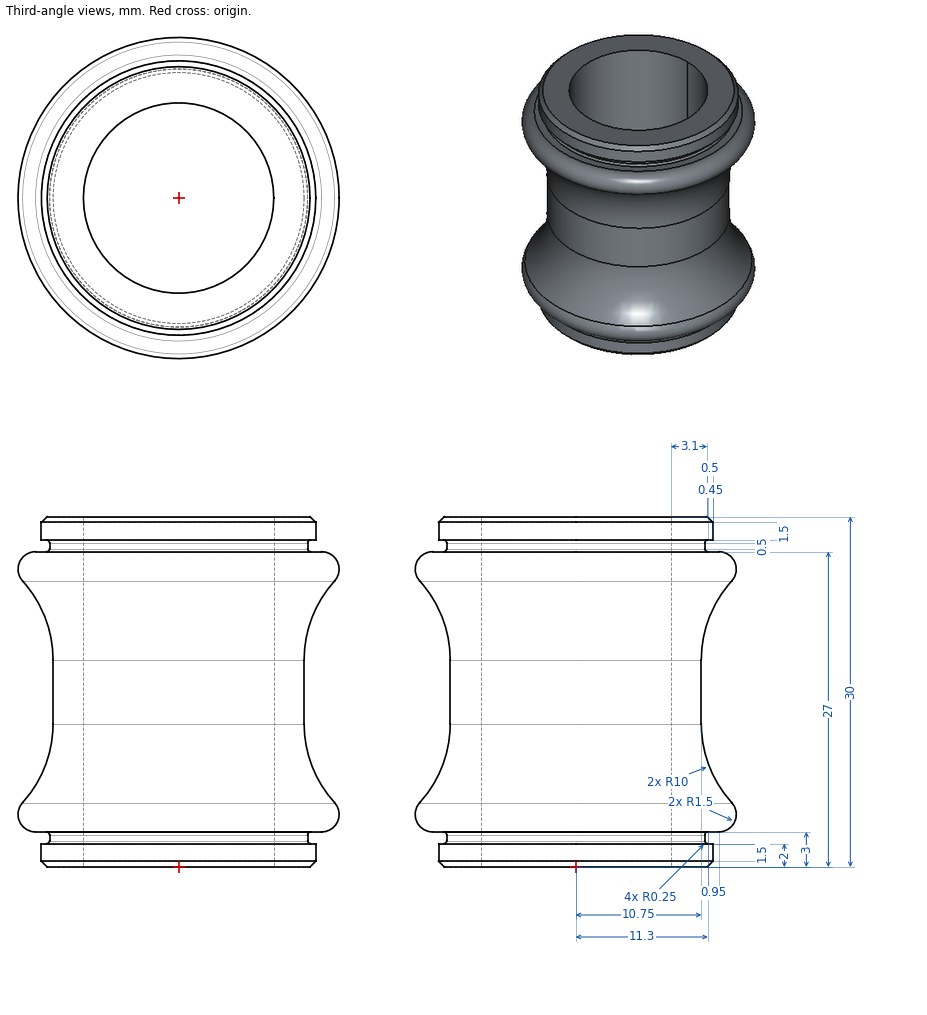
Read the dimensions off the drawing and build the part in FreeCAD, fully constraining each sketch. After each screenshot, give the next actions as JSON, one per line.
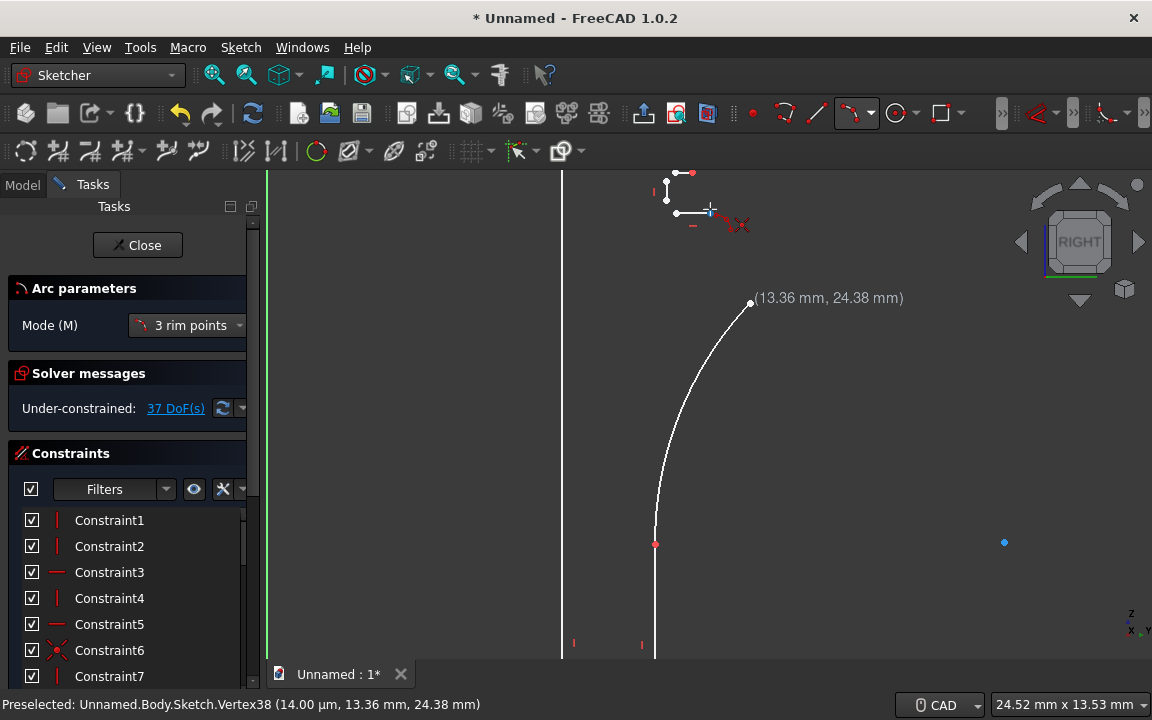
{"action": "left_click", "coordinate": [710, 213]}
{"action": "left_click", "coordinate": [760, 241]}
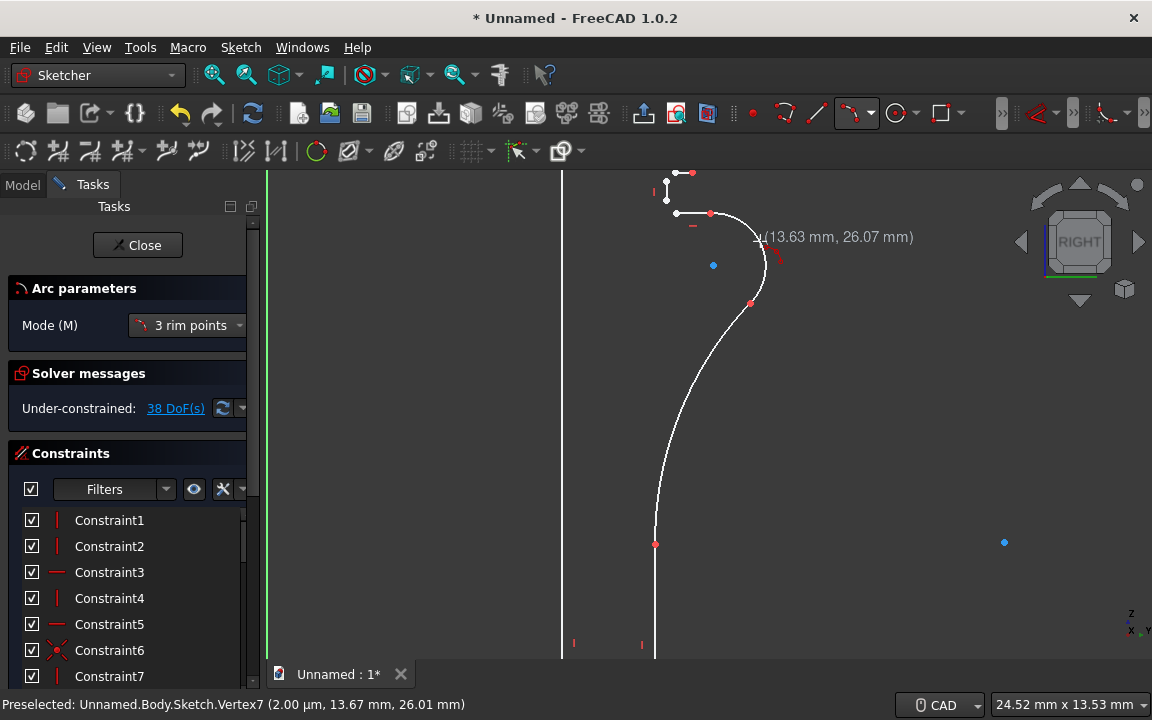
{"action": "scroll", "coordinate": [676, 208], "scroll_direction": "up", "scroll_amount": 2}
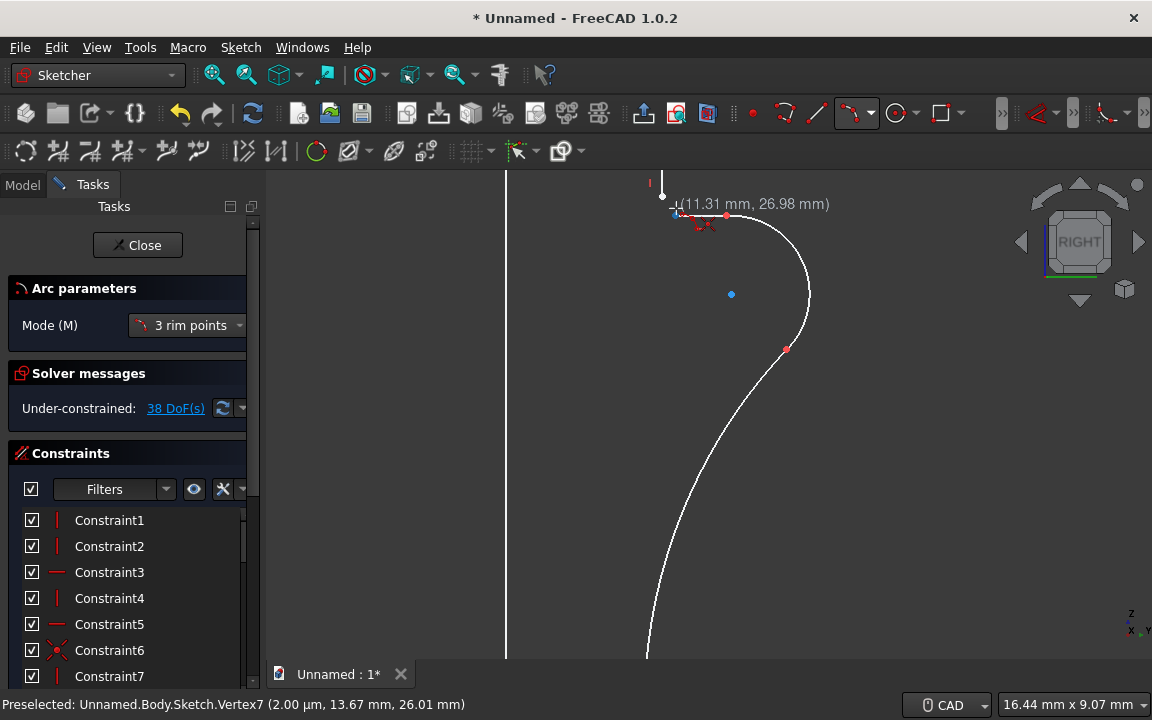
{"action": "left_click", "coordinate": [676, 216]}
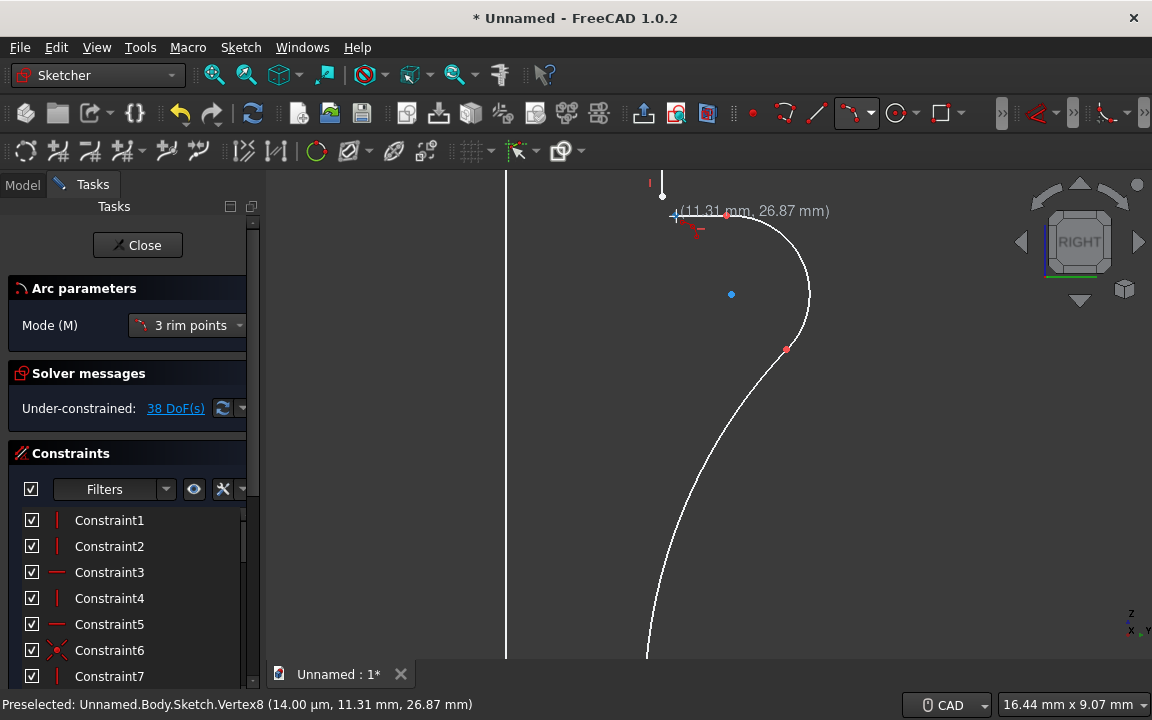
{"action": "scroll", "coordinate": [693, 303], "scroll_direction": "down", "scroll_amount": 8}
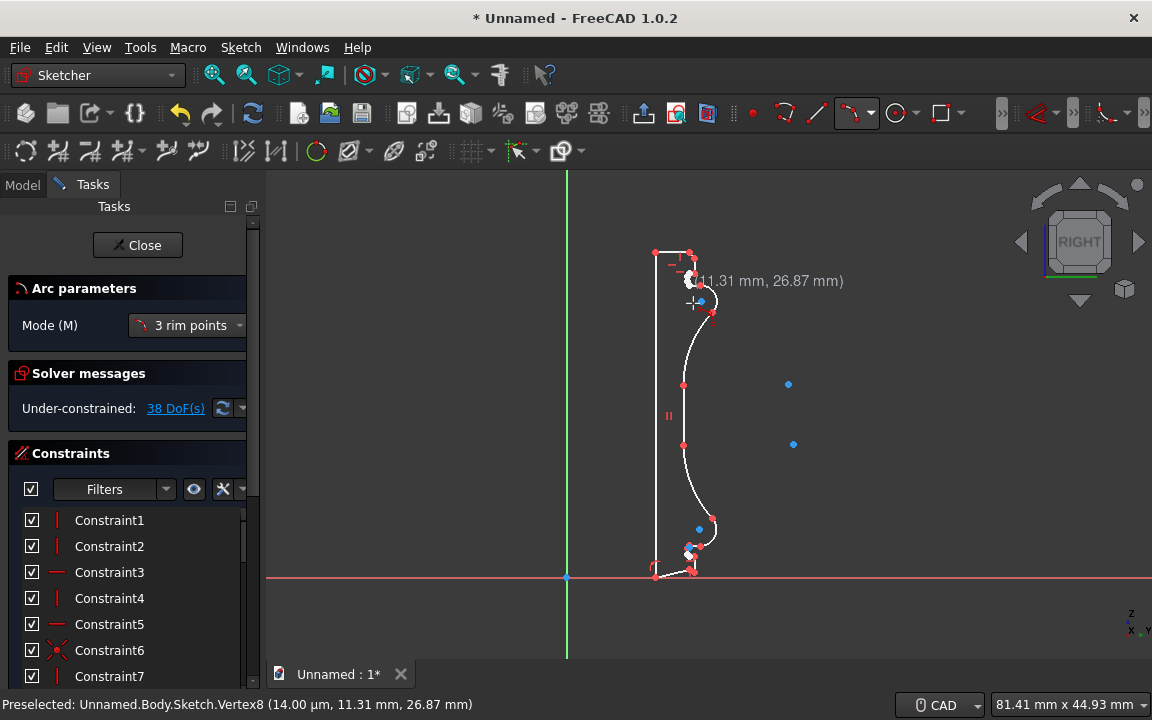
{"action": "scroll", "coordinate": [687, 281], "scroll_direction": "up", "scroll_amount": 9}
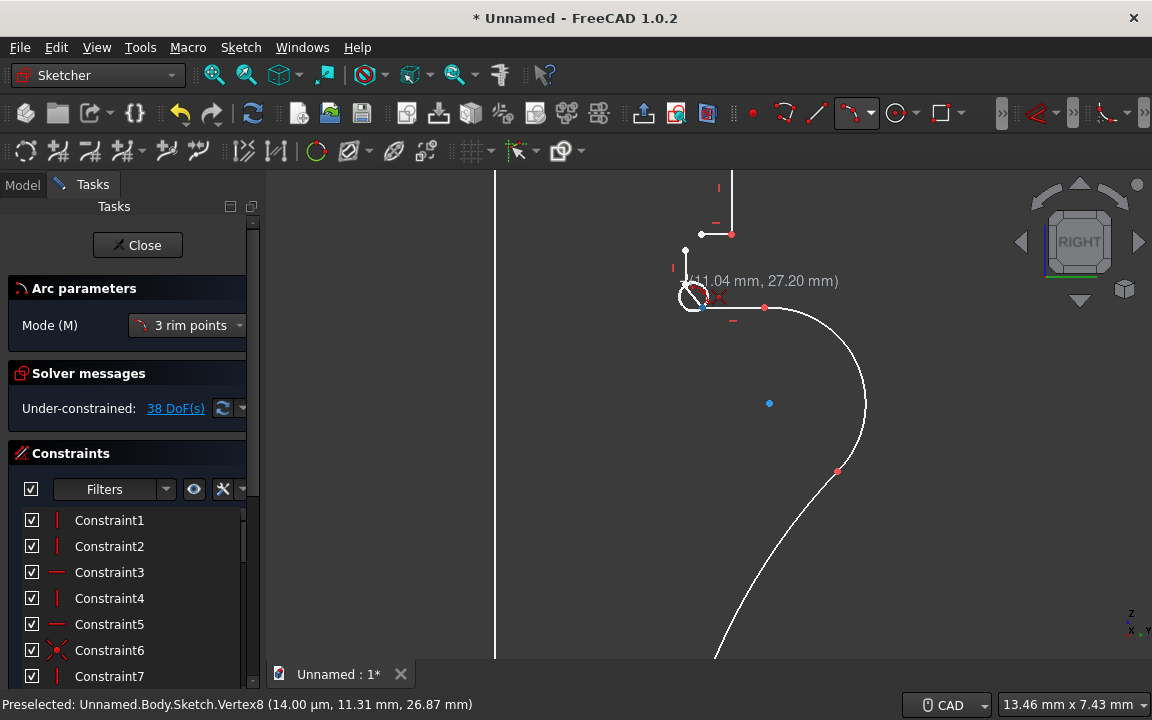
{"action": "left_click", "coordinate": [686, 284]}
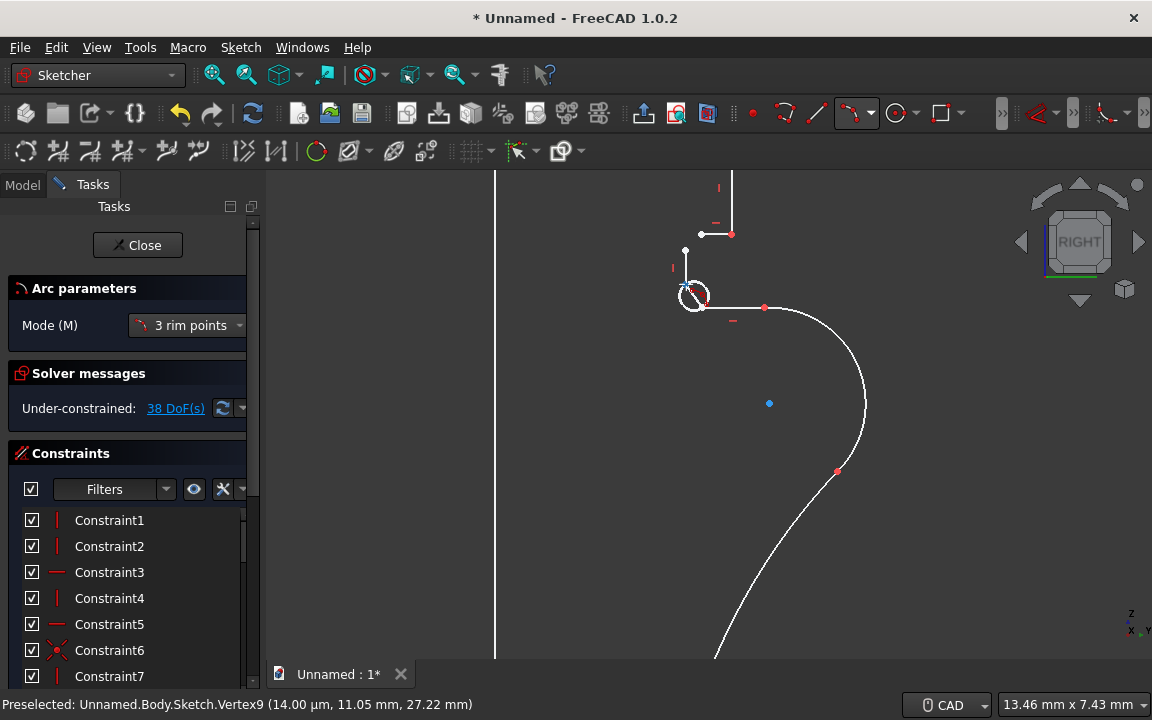
{"action": "scroll", "coordinate": [690, 294], "scroll_direction": "up", "scroll_amount": 6}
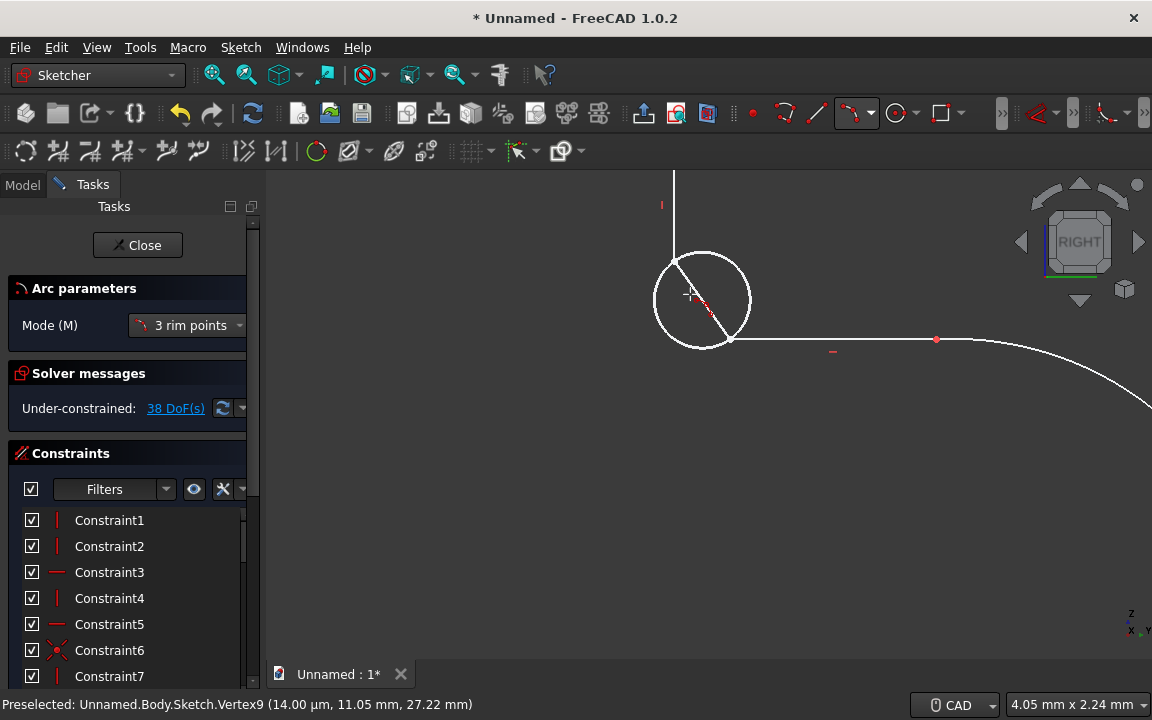
{"action": "left_click", "coordinate": [689, 294]}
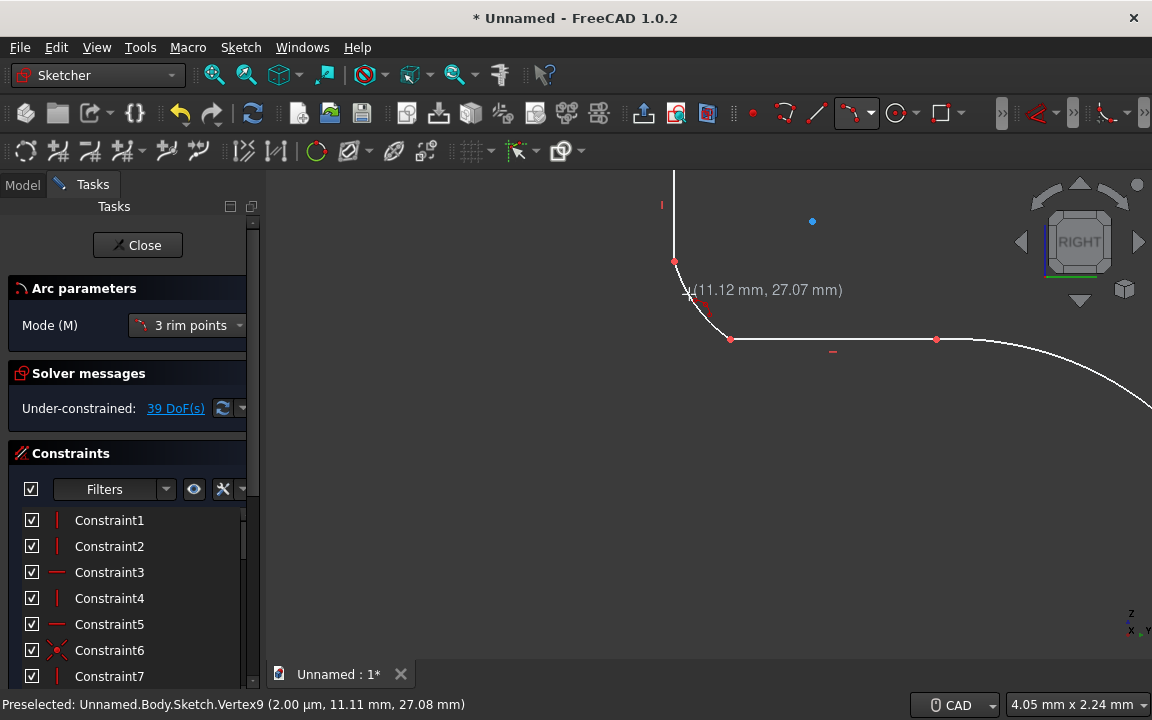
{"action": "scroll", "coordinate": [687, 283], "scroll_direction": "down", "scroll_amount": 15}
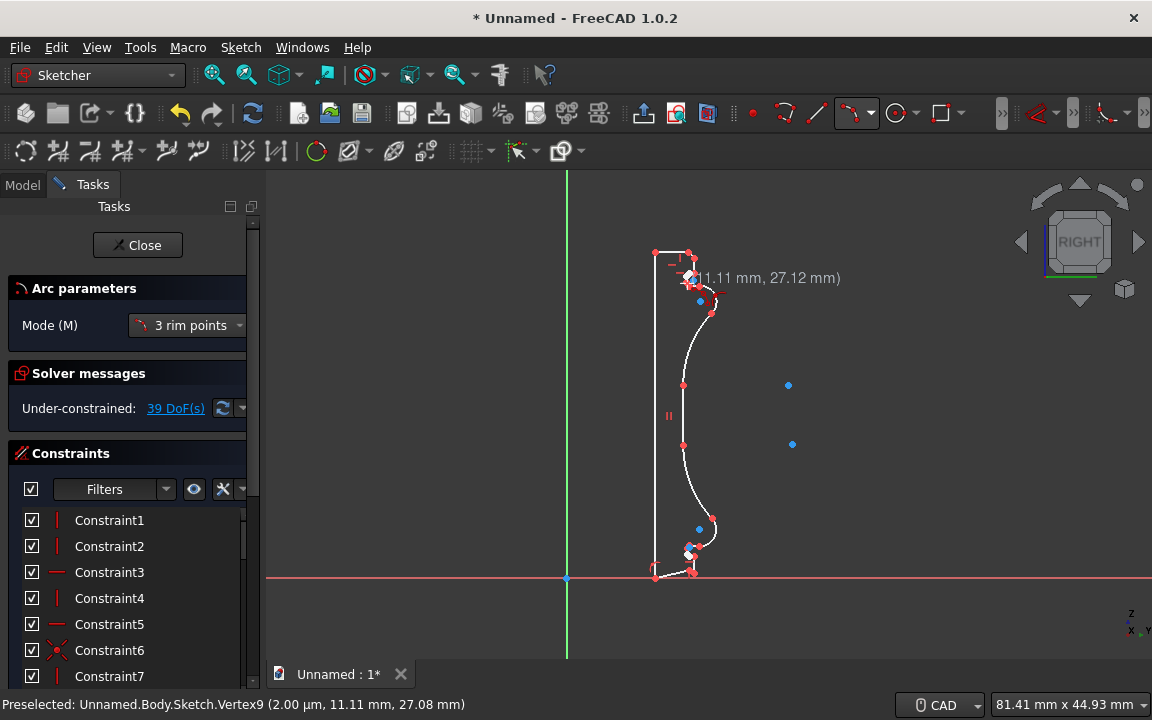
{"action": "scroll", "coordinate": [687, 276], "scroll_direction": "up", "scroll_amount": 9}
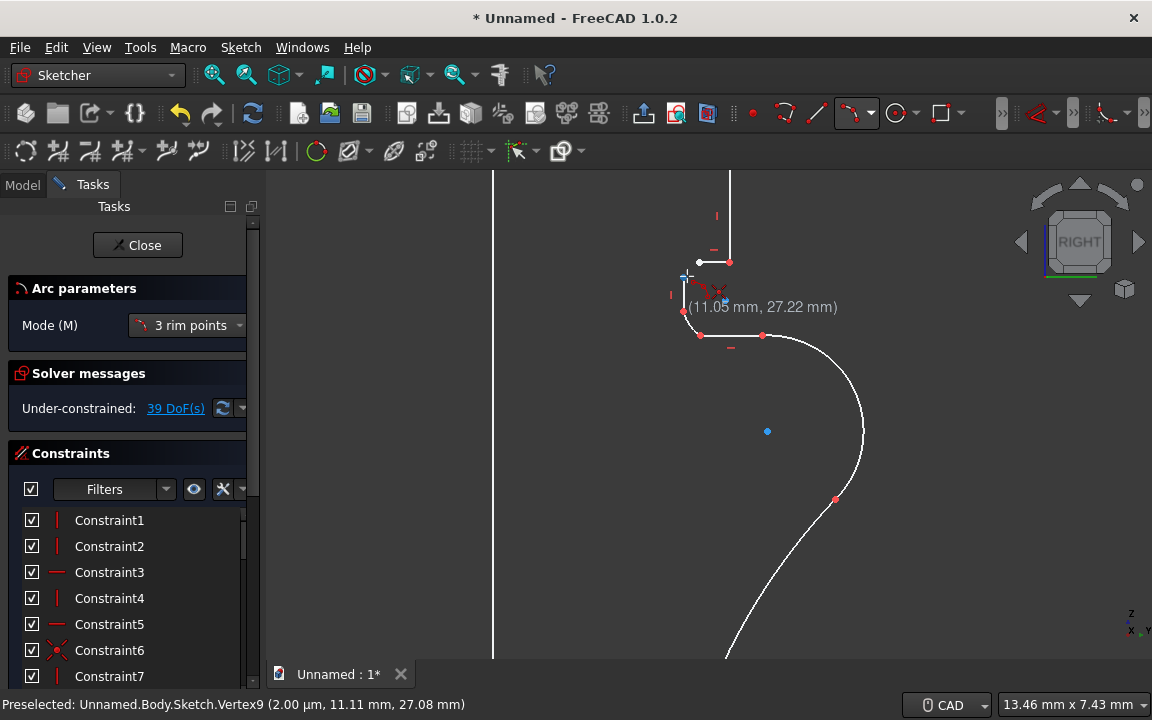
{"action": "left_click", "coordinate": [684, 278]}
{"action": "left_click", "coordinate": [699, 262]}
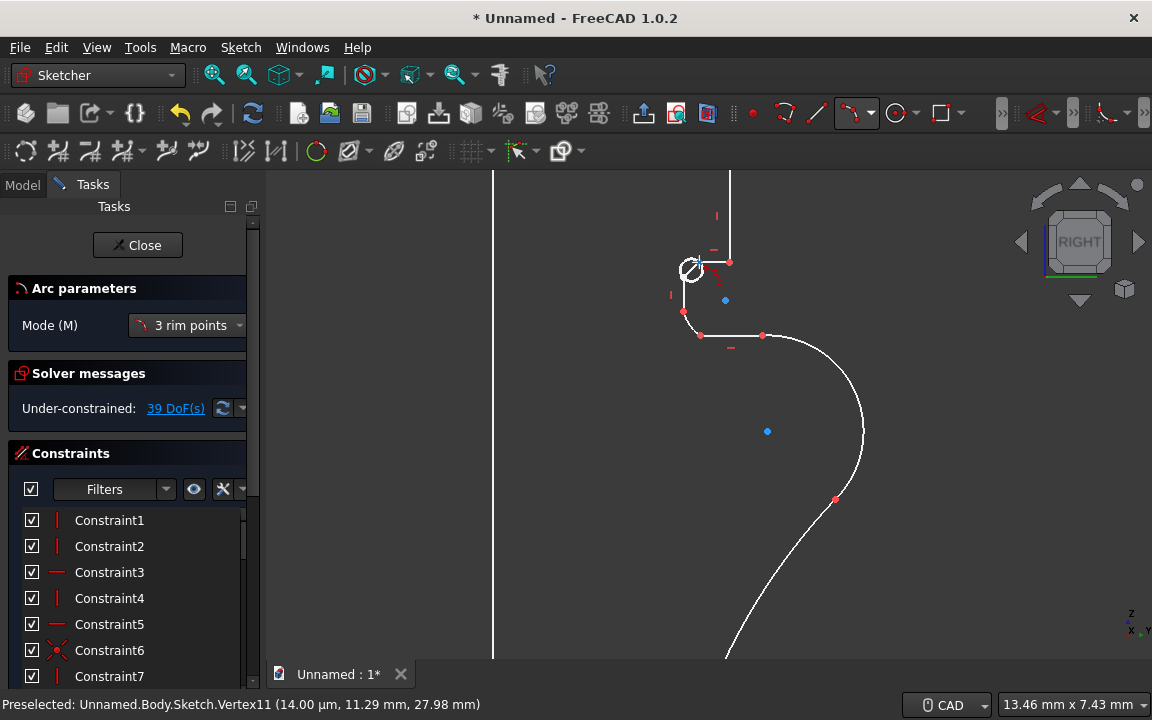
{"action": "scroll", "coordinate": [688, 266], "scroll_direction": "up", "scroll_amount": 6}